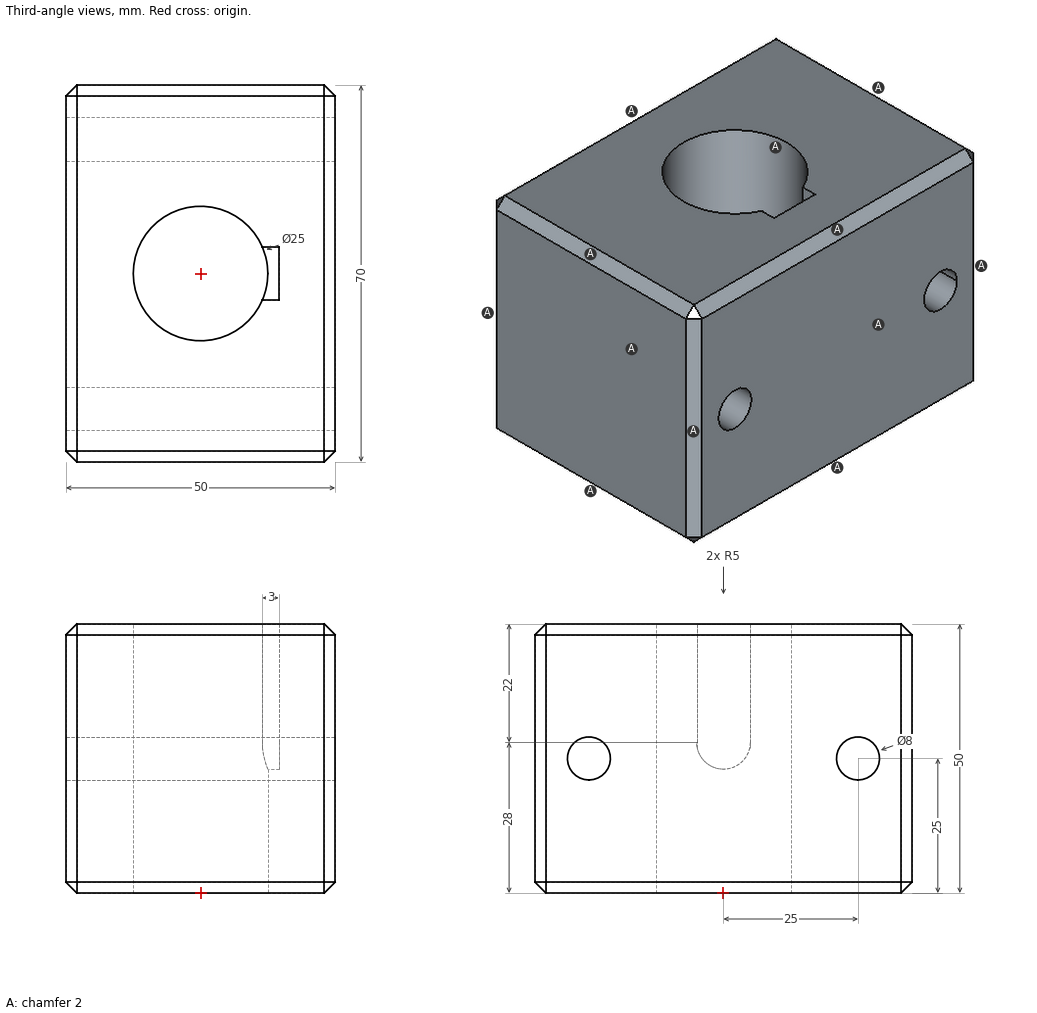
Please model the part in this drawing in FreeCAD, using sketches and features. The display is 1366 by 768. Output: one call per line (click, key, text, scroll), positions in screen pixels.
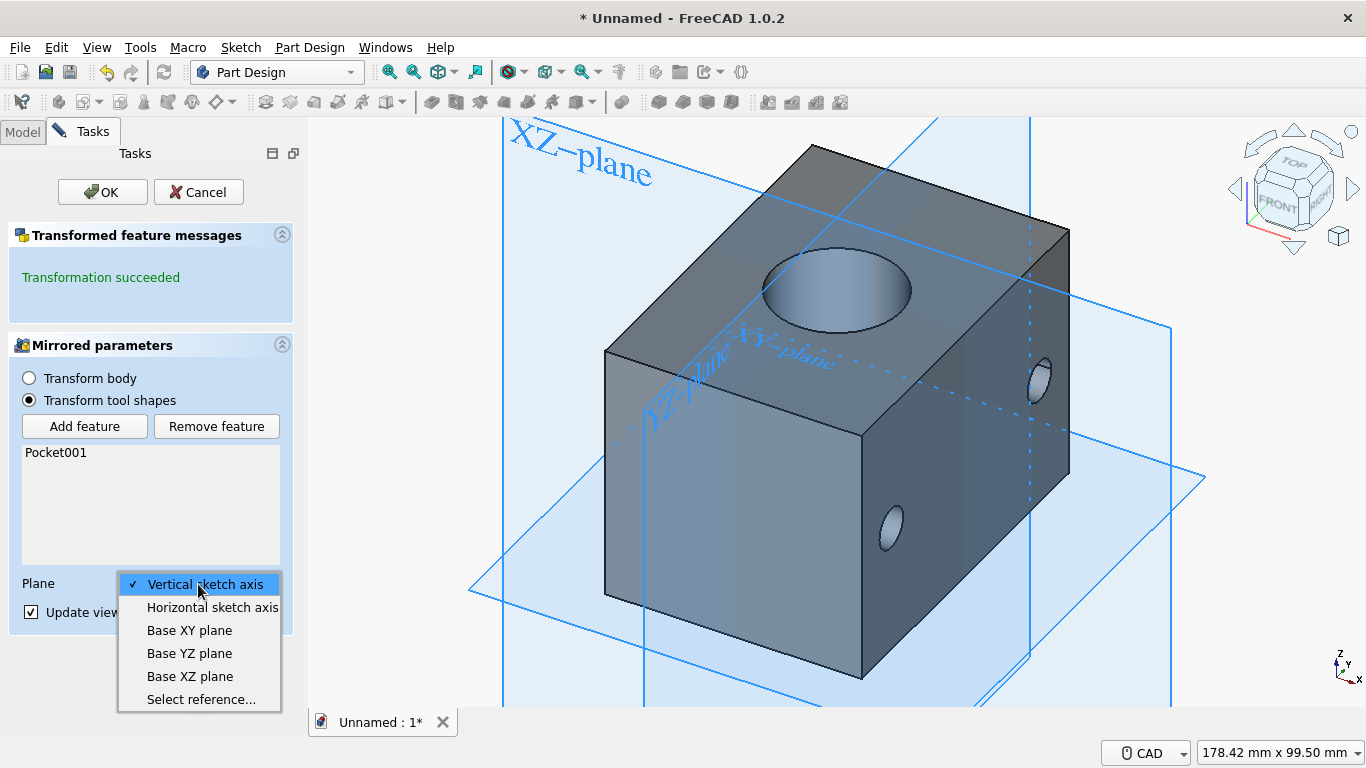
click(198, 676)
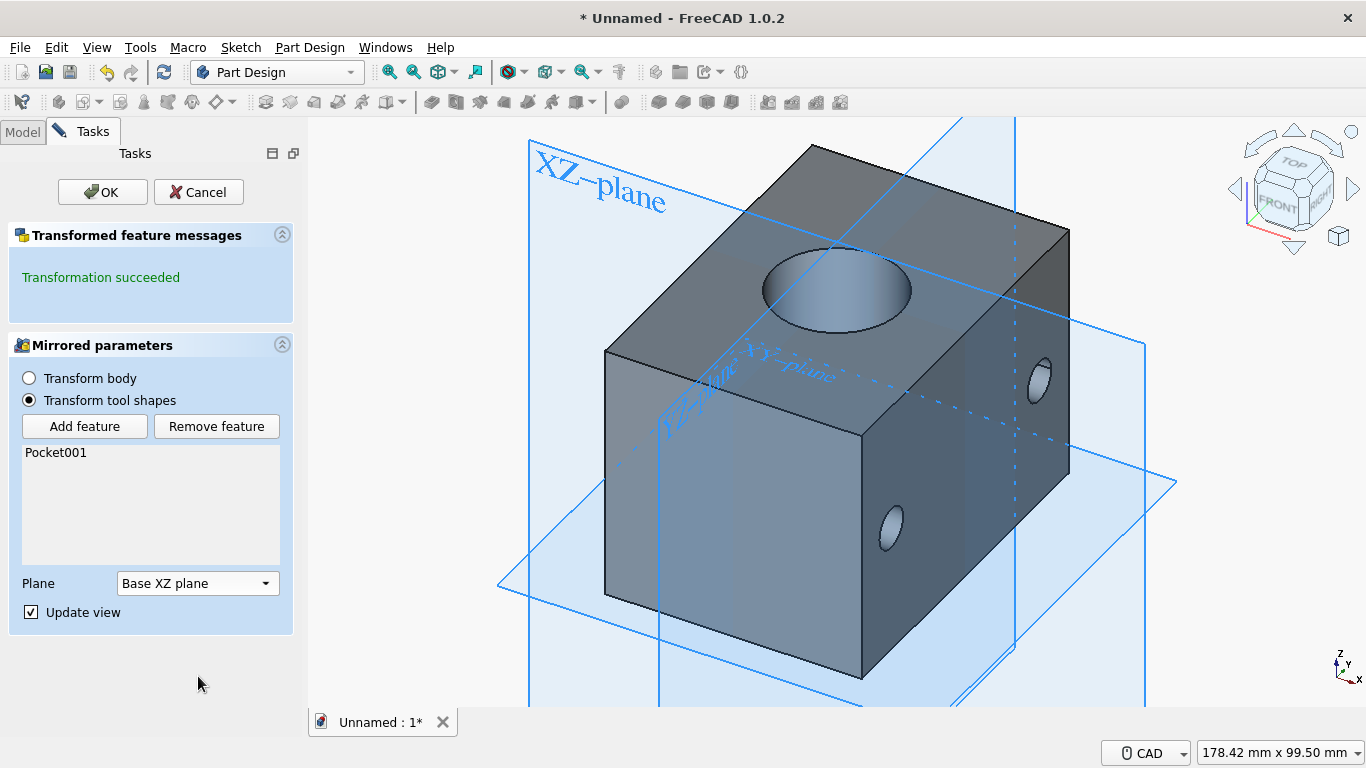
click(103, 192)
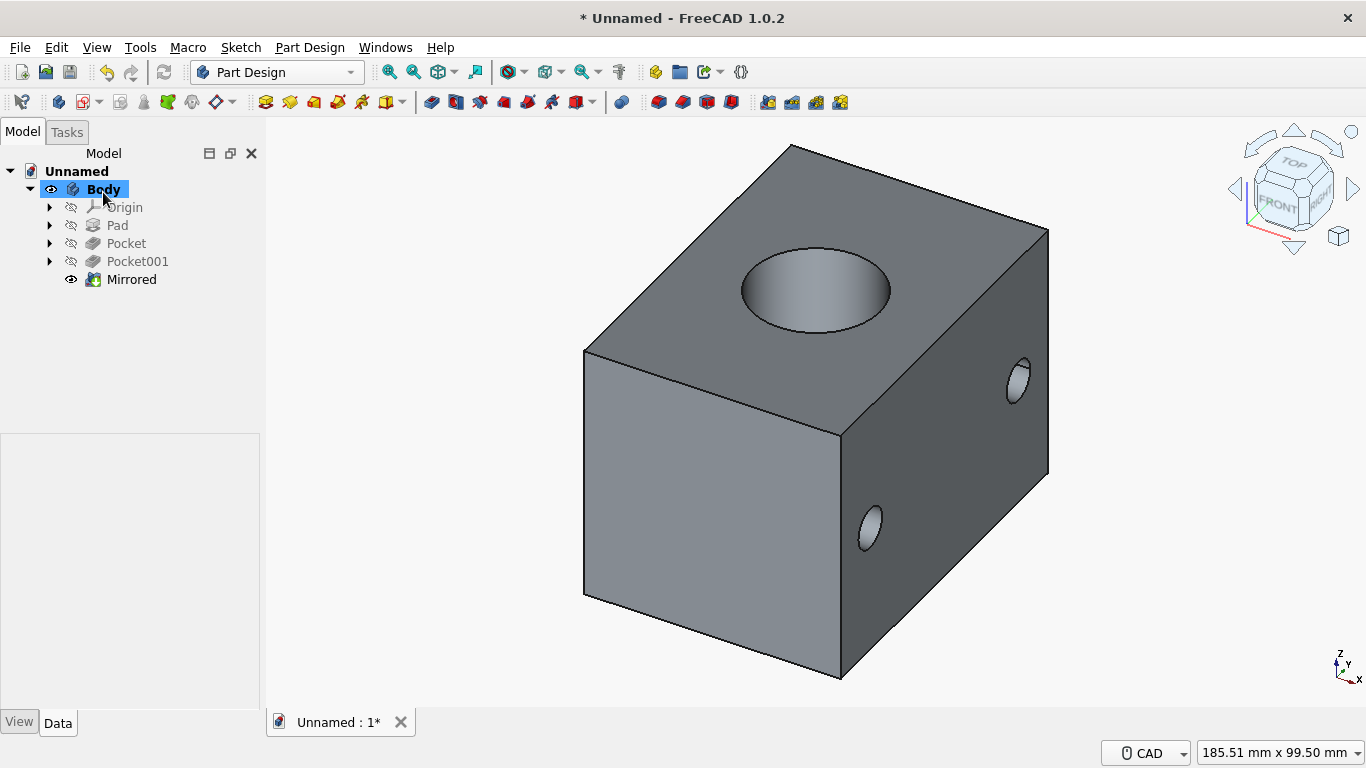
click(712, 514)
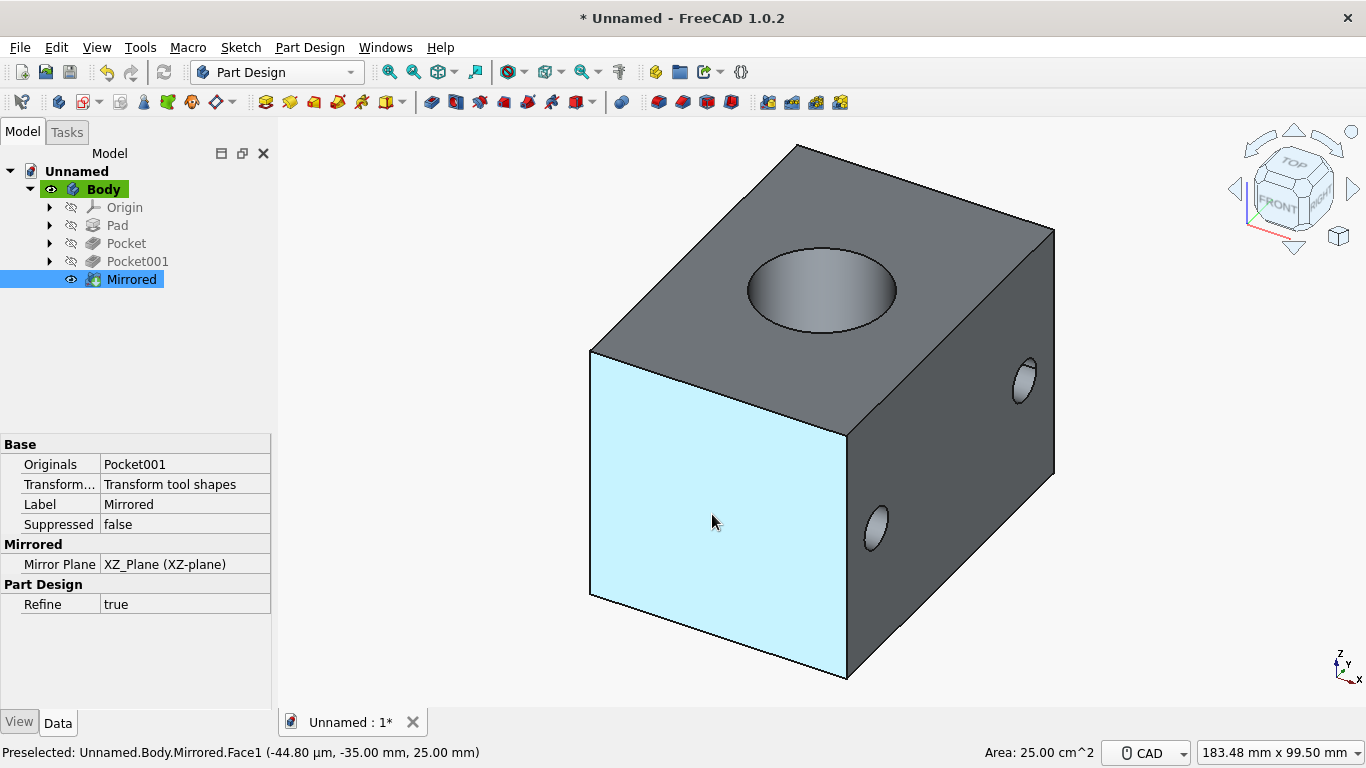
click(950, 332, ctrl)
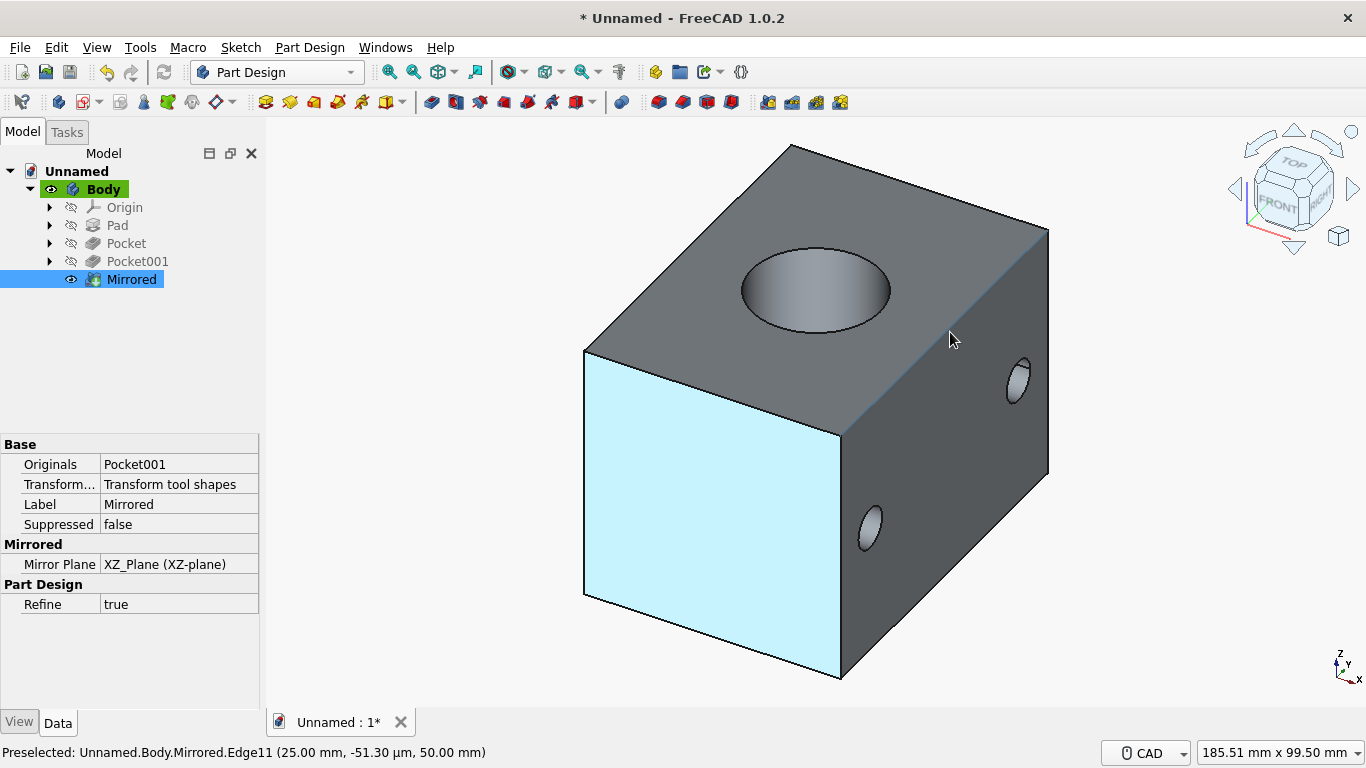
key(0)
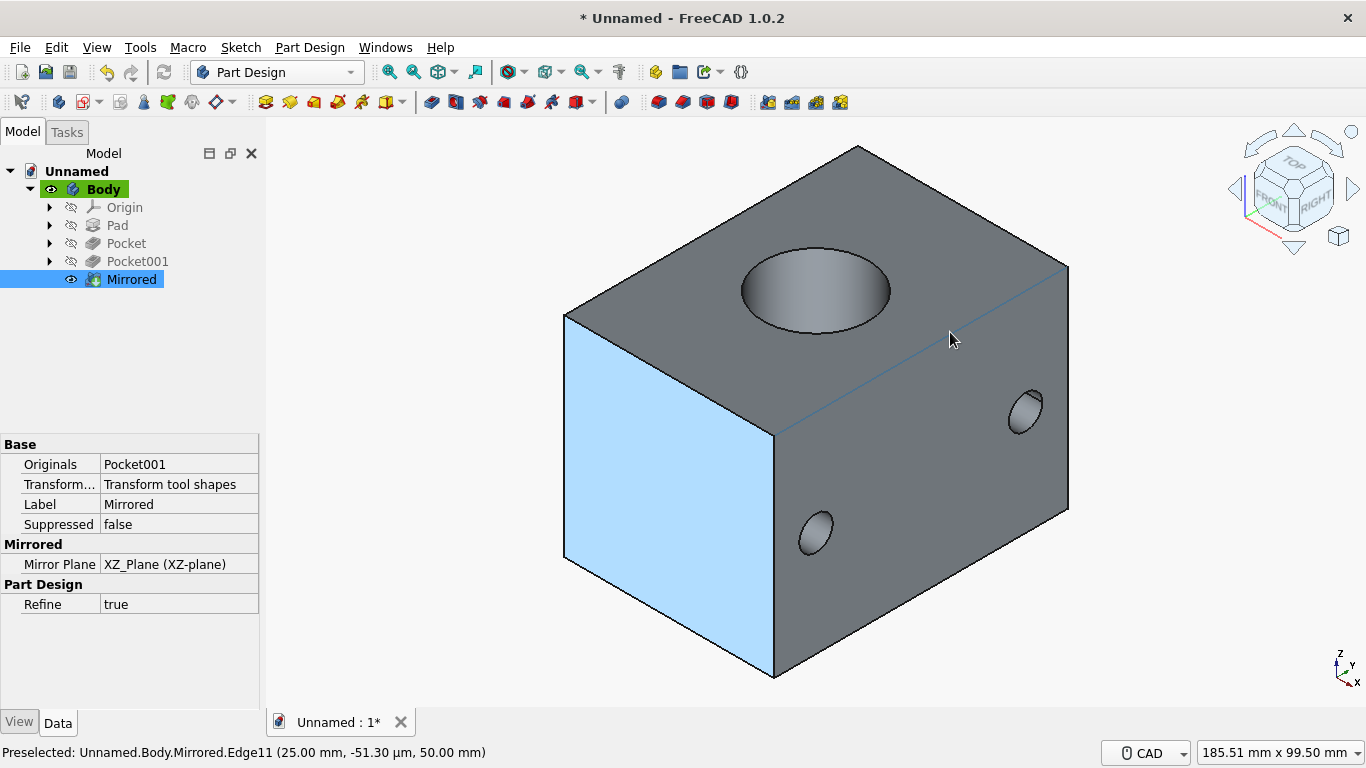
key(2)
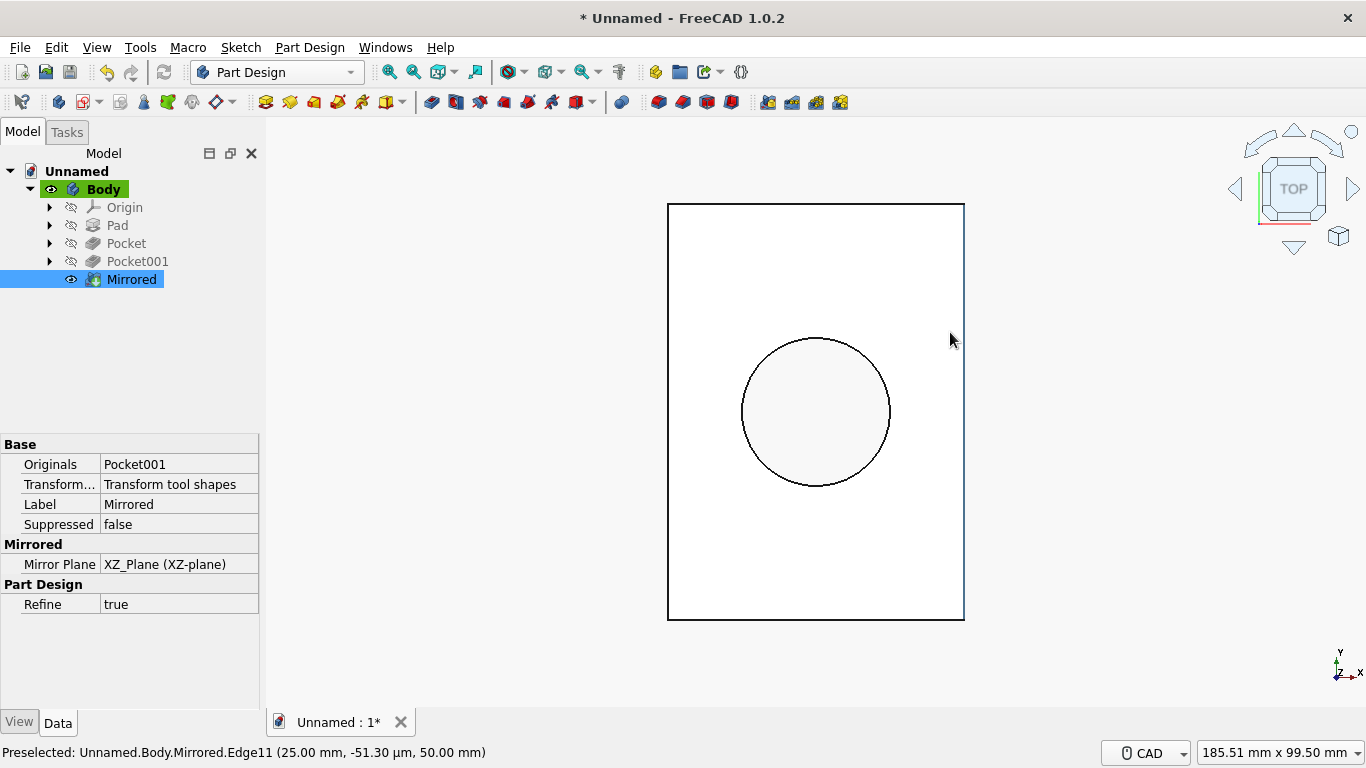
click(668, 411, ctrl)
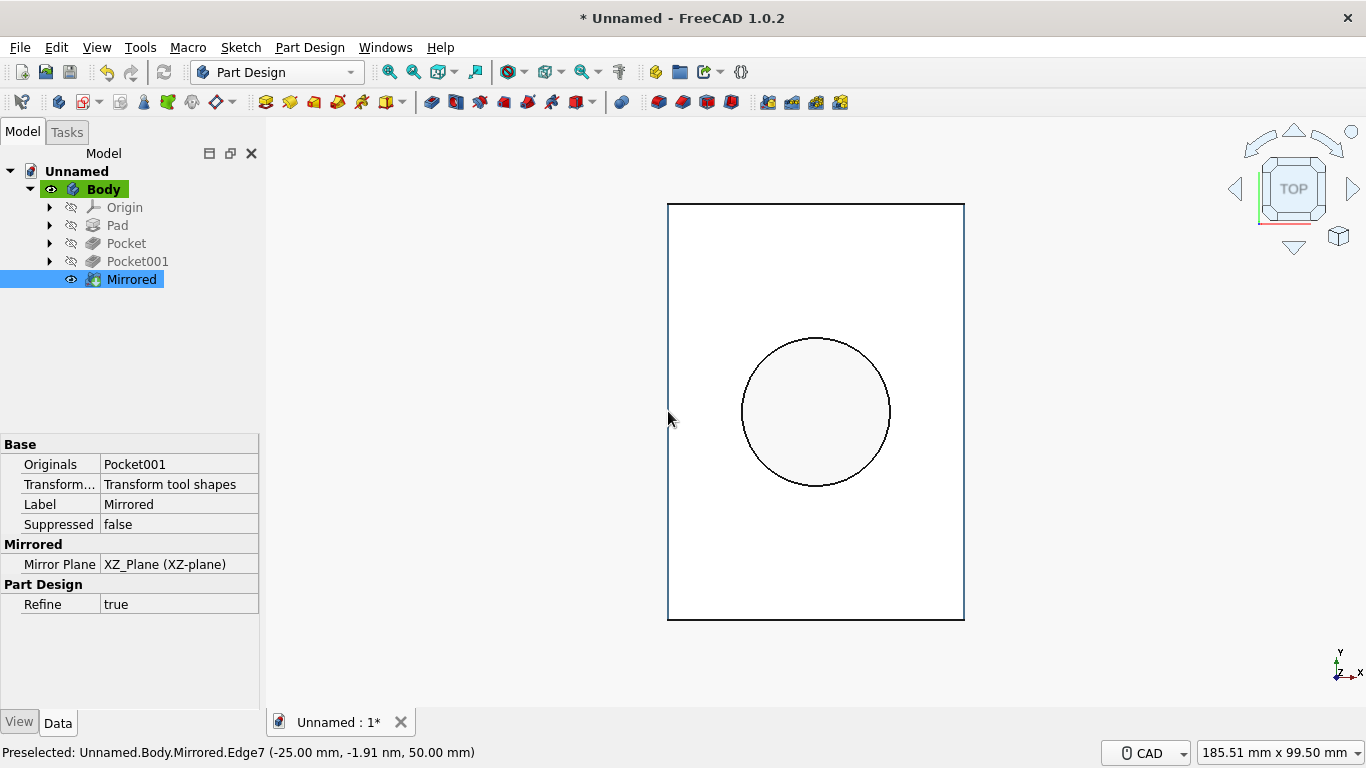
key(1)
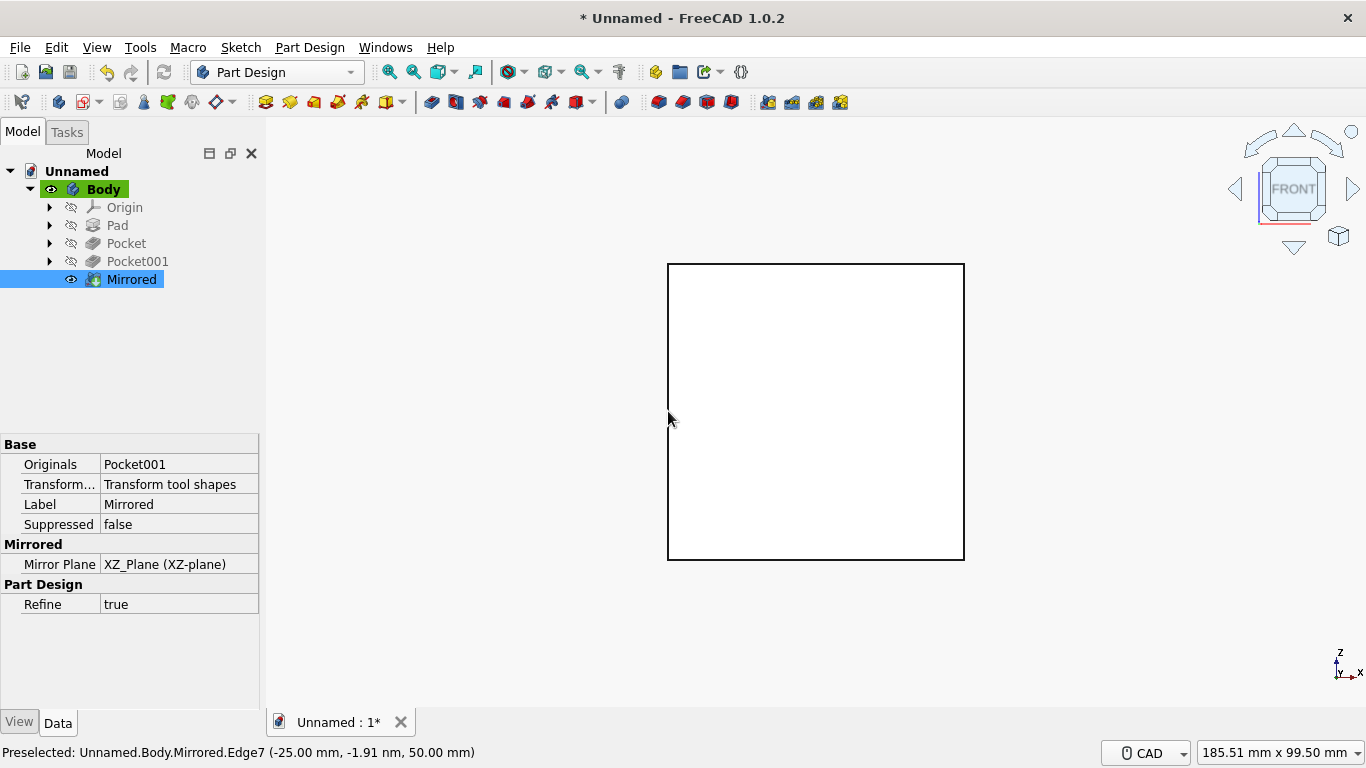
key(3)